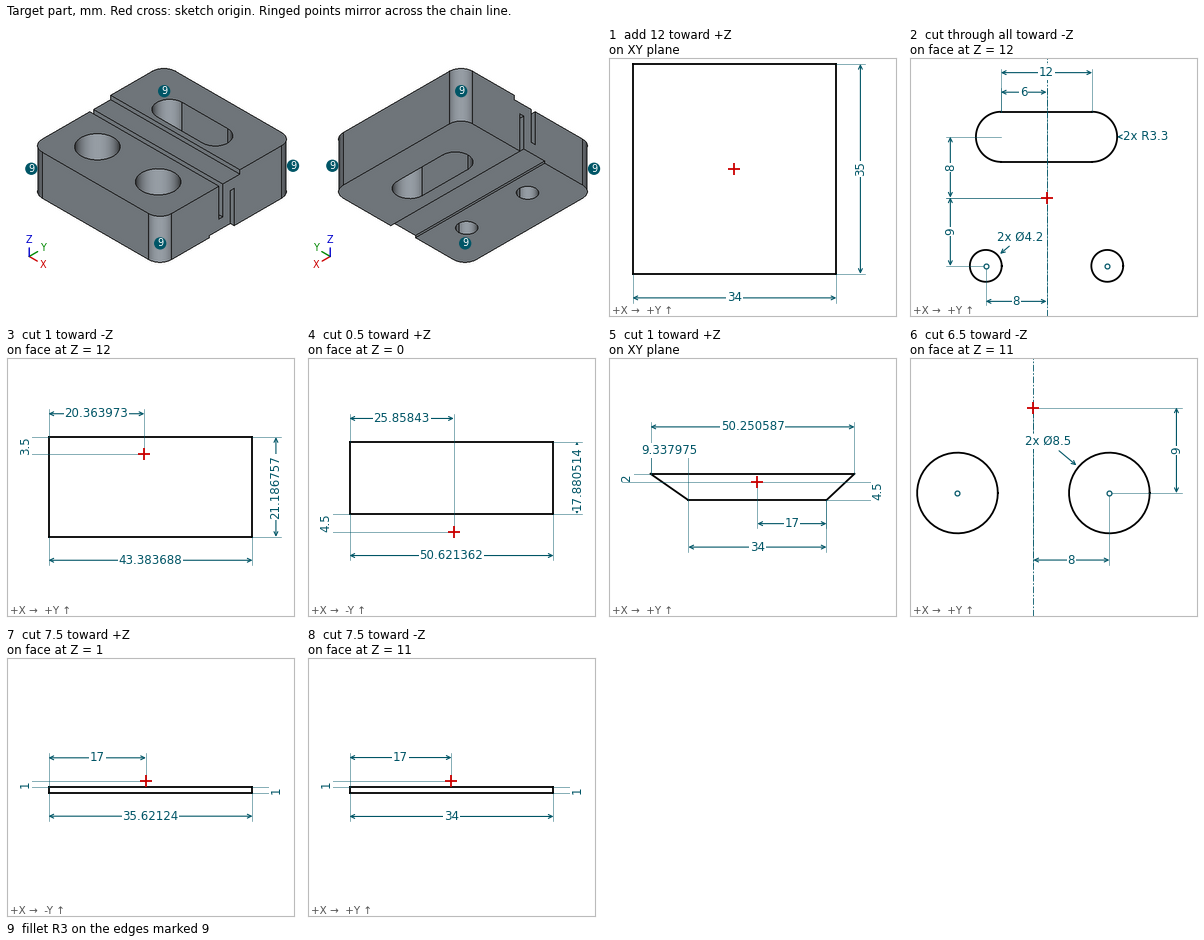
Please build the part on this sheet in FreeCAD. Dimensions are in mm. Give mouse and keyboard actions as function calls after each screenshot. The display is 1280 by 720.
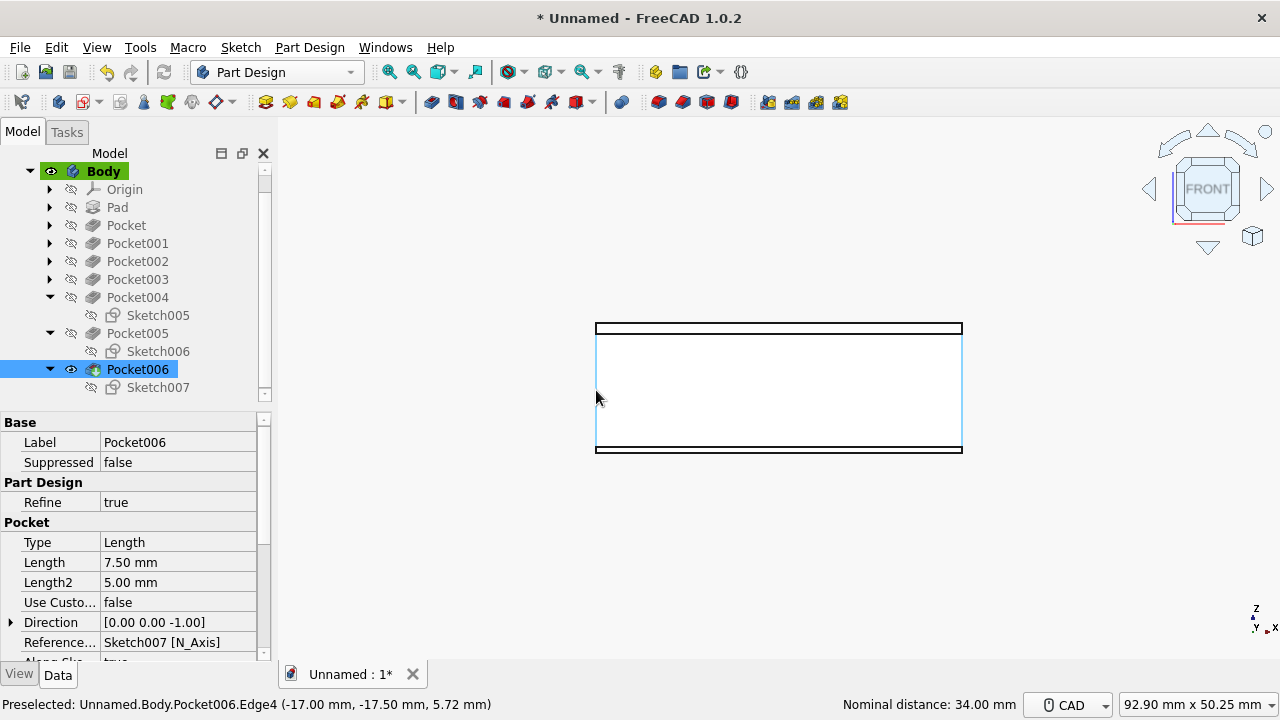
key(3)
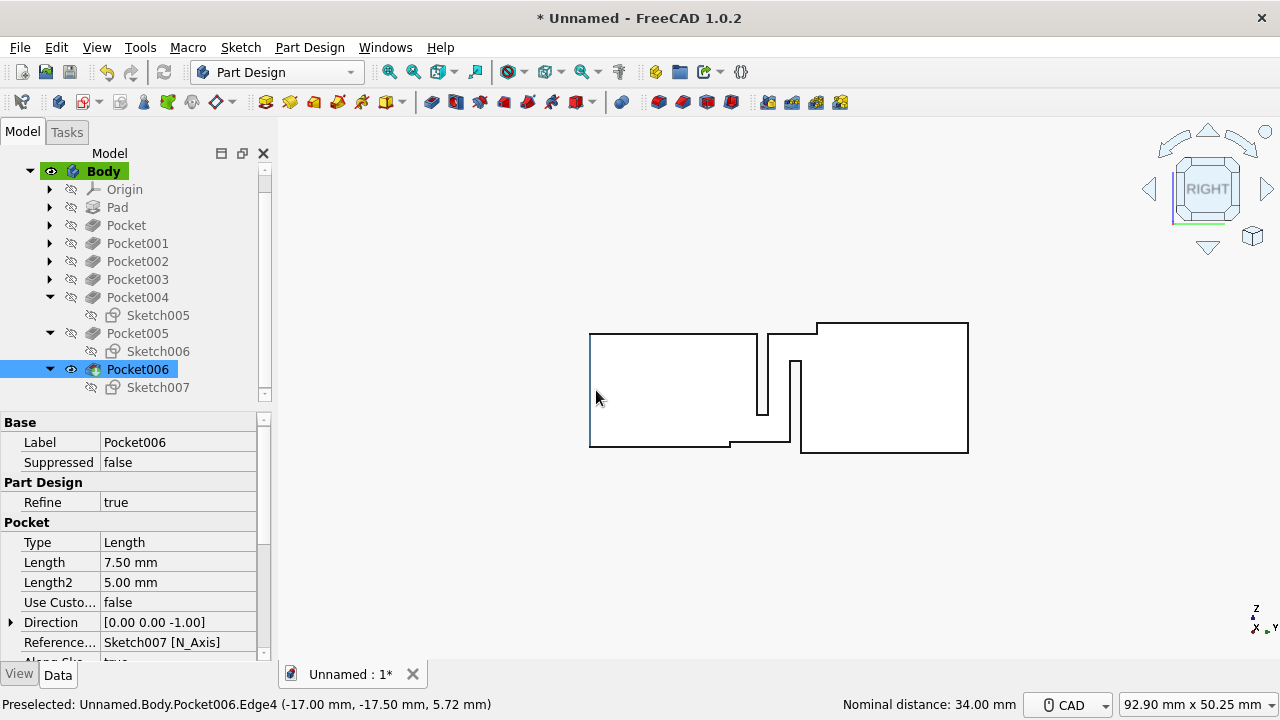
key(v)
key(f)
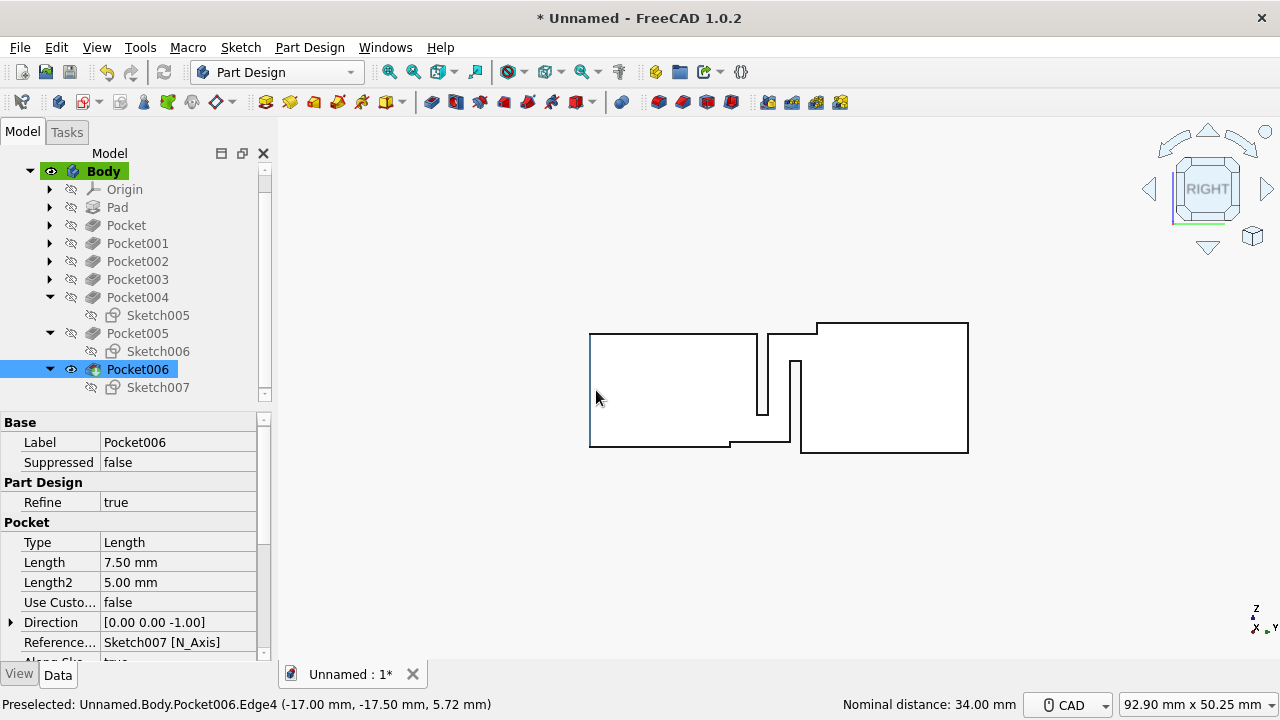
click(968, 387, ctrl)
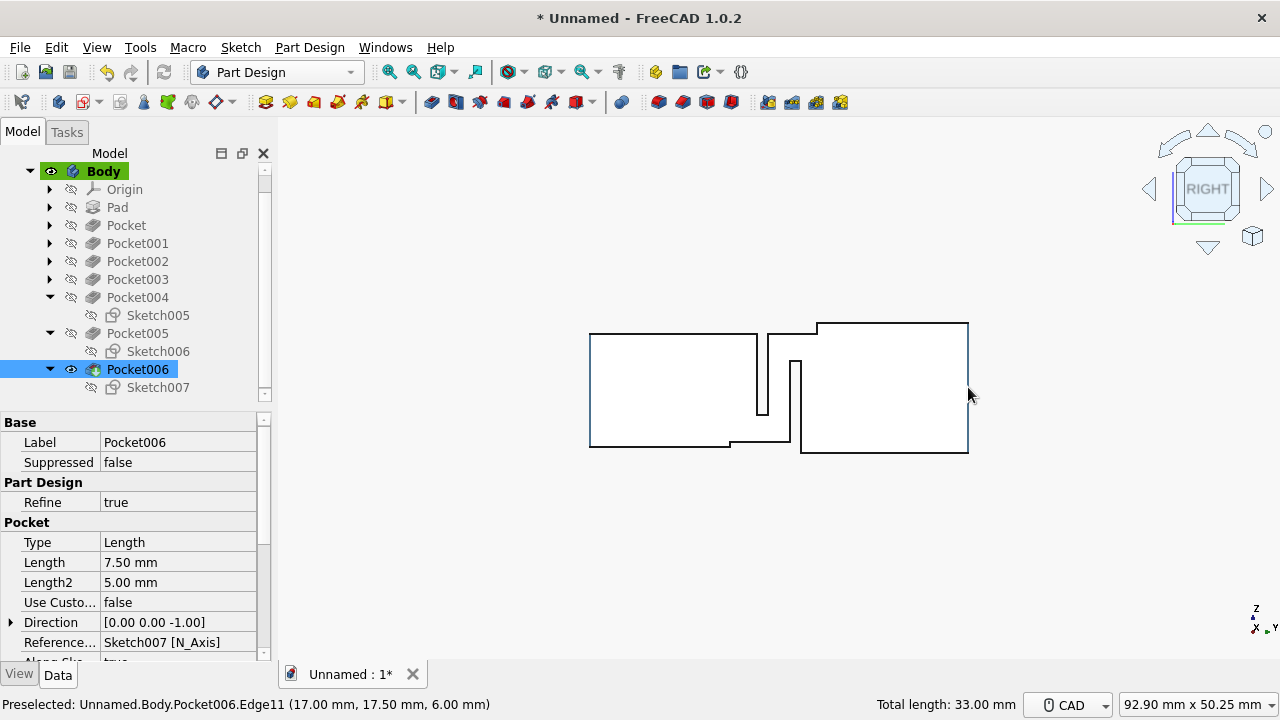
key(5)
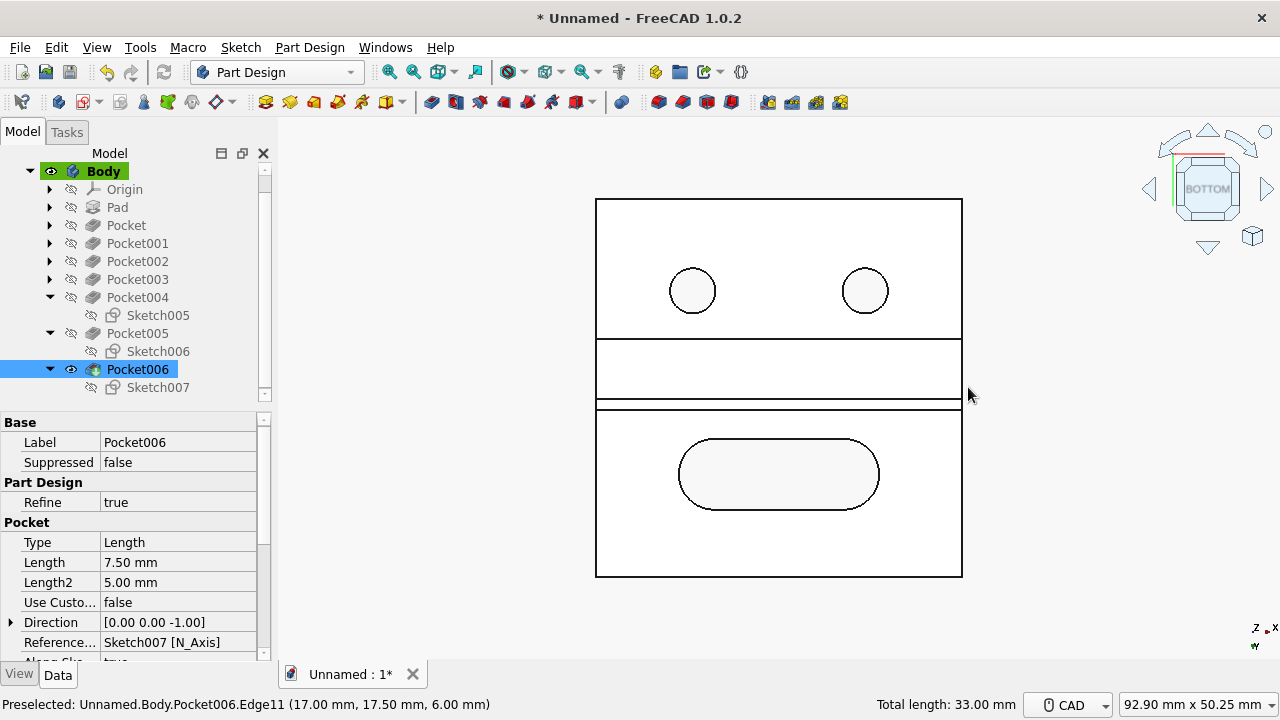
key(4)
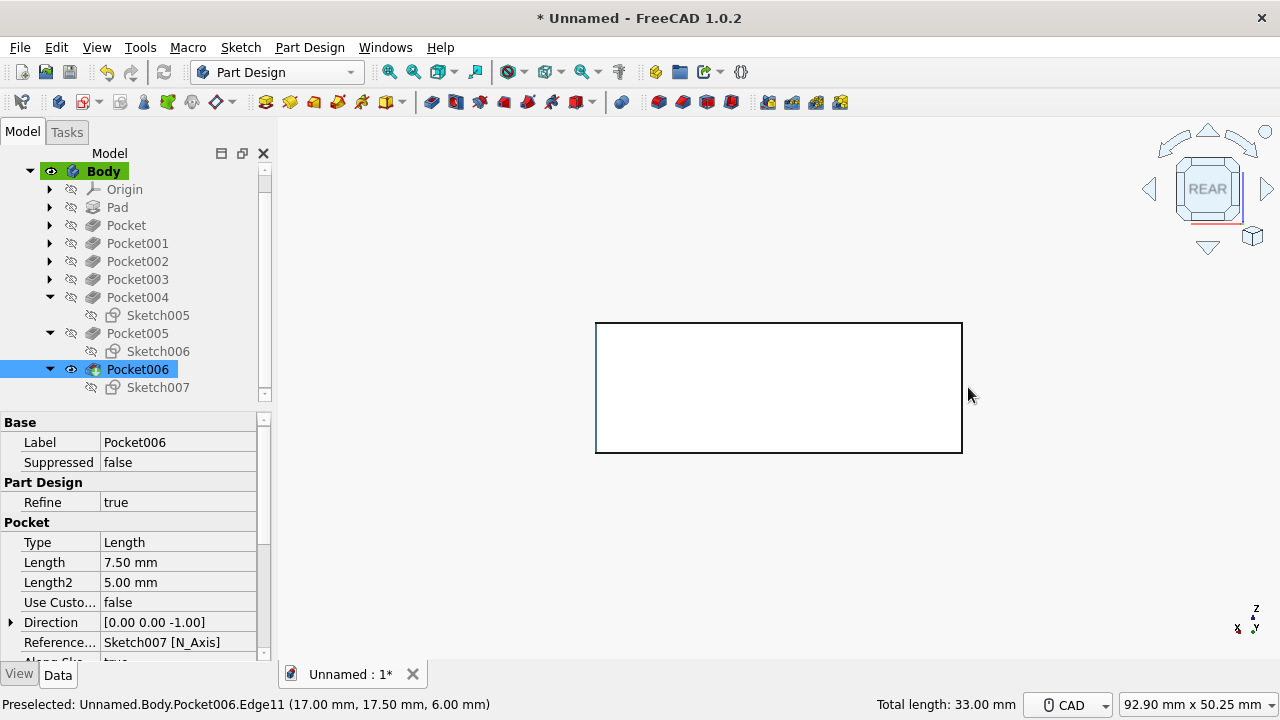
key(v)
key(f)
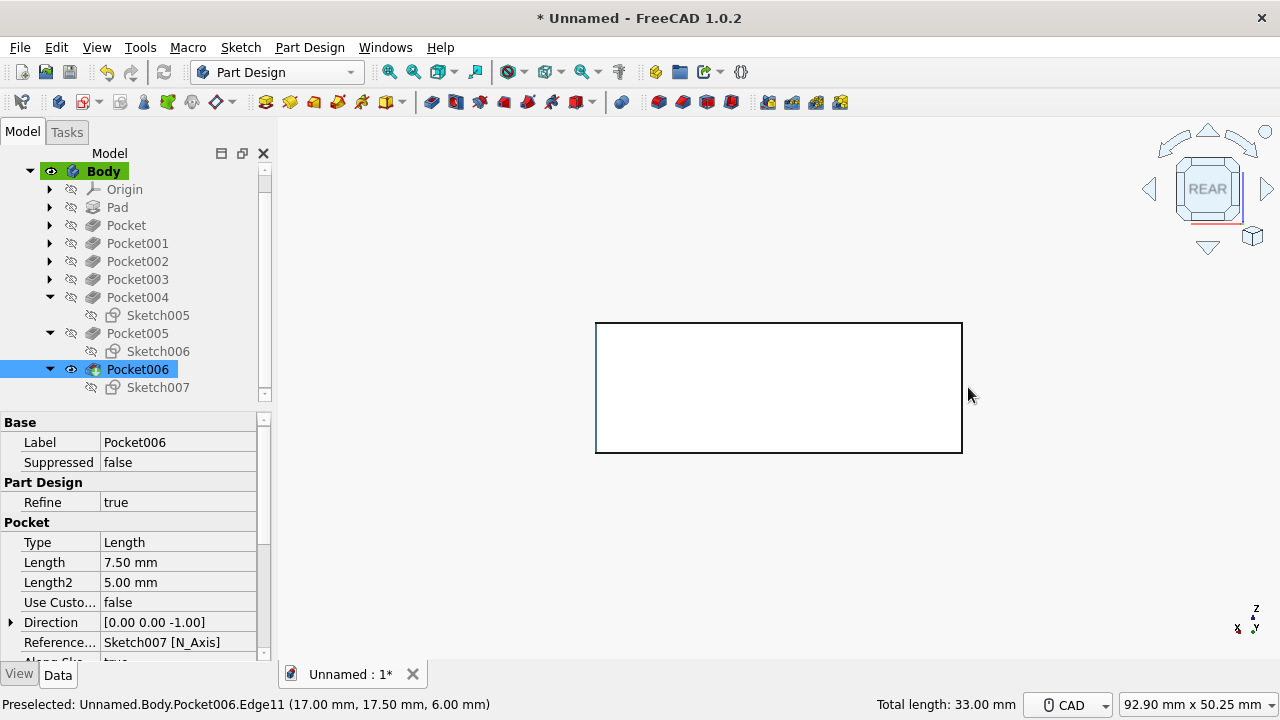
click(962, 387, ctrl)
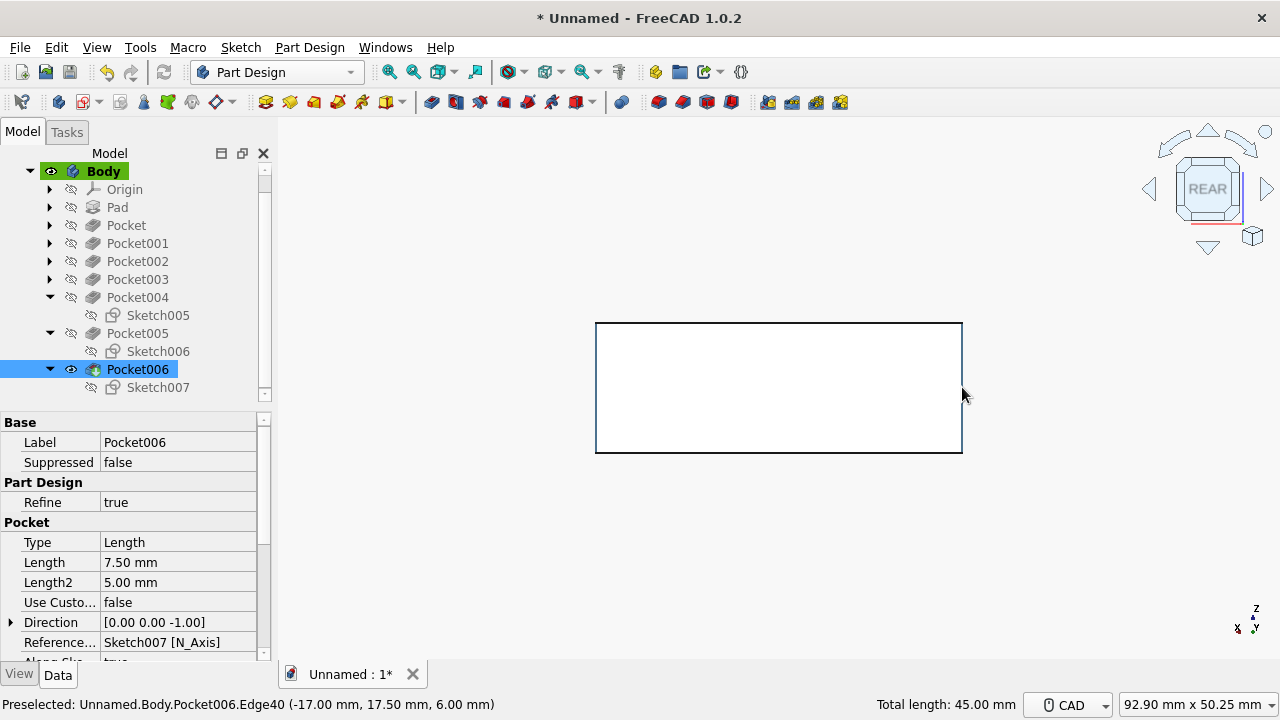
click(660, 102)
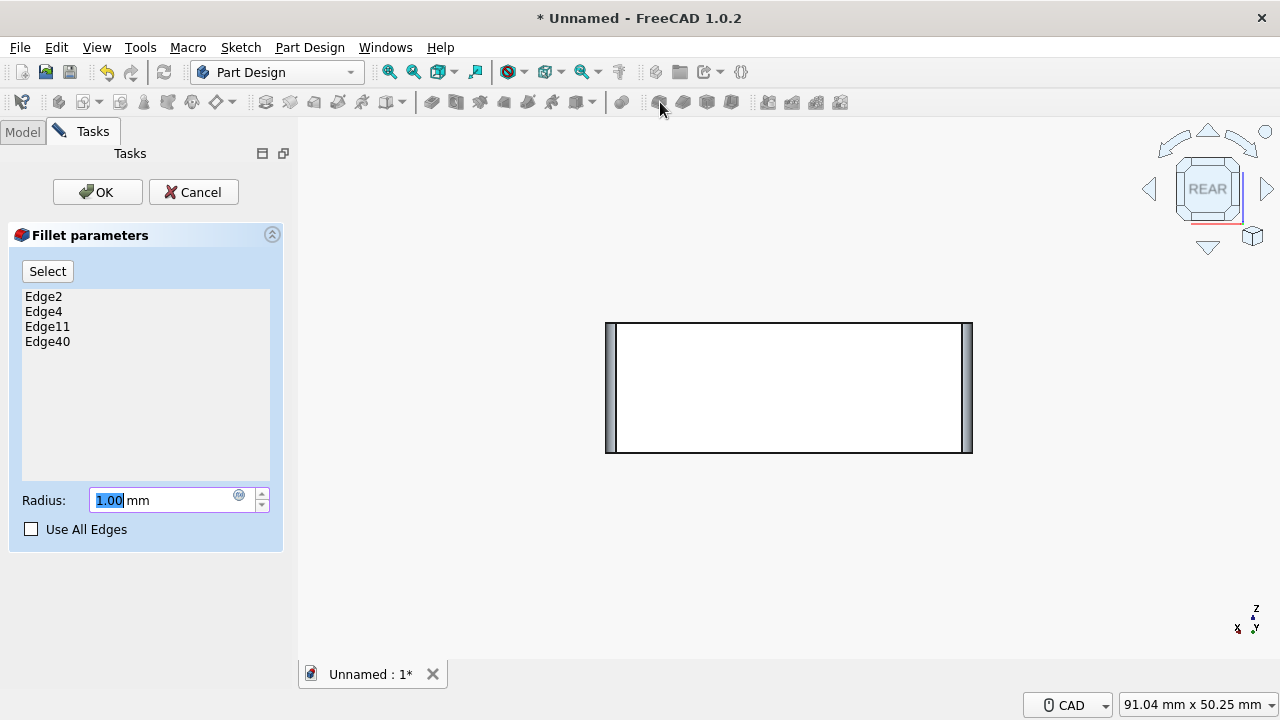
text(3)
key(Tab)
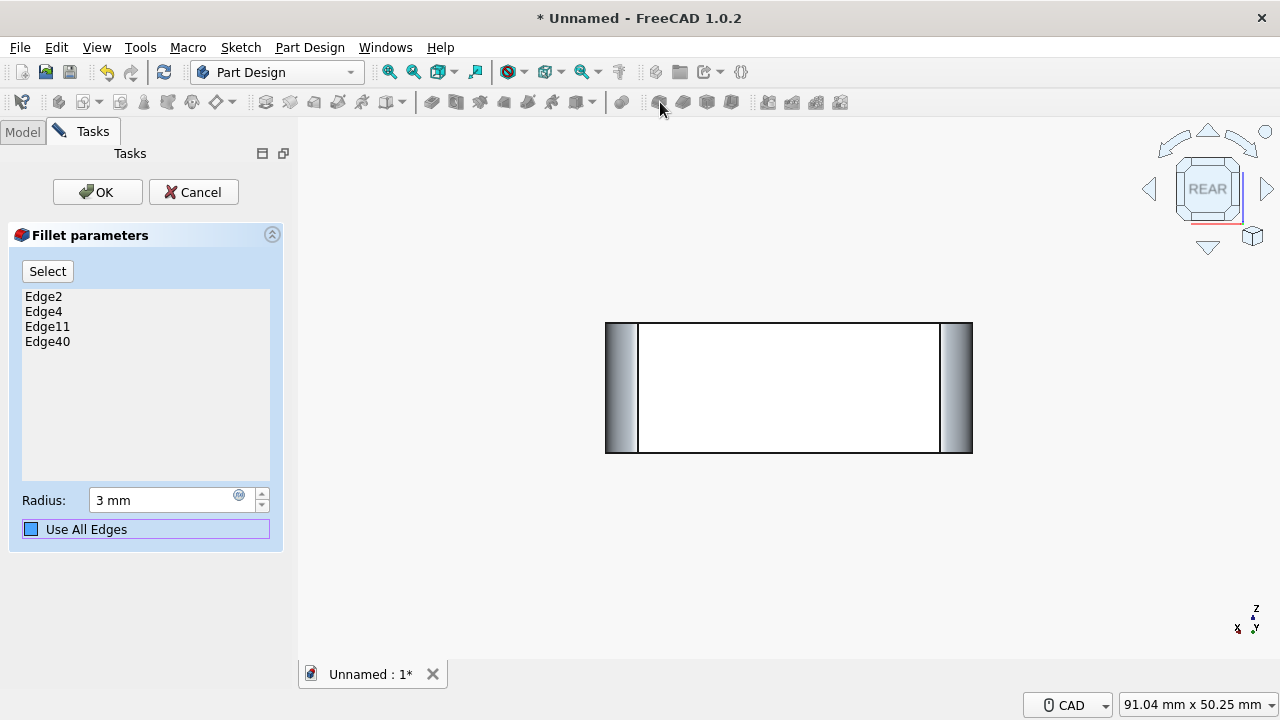
click(98, 192)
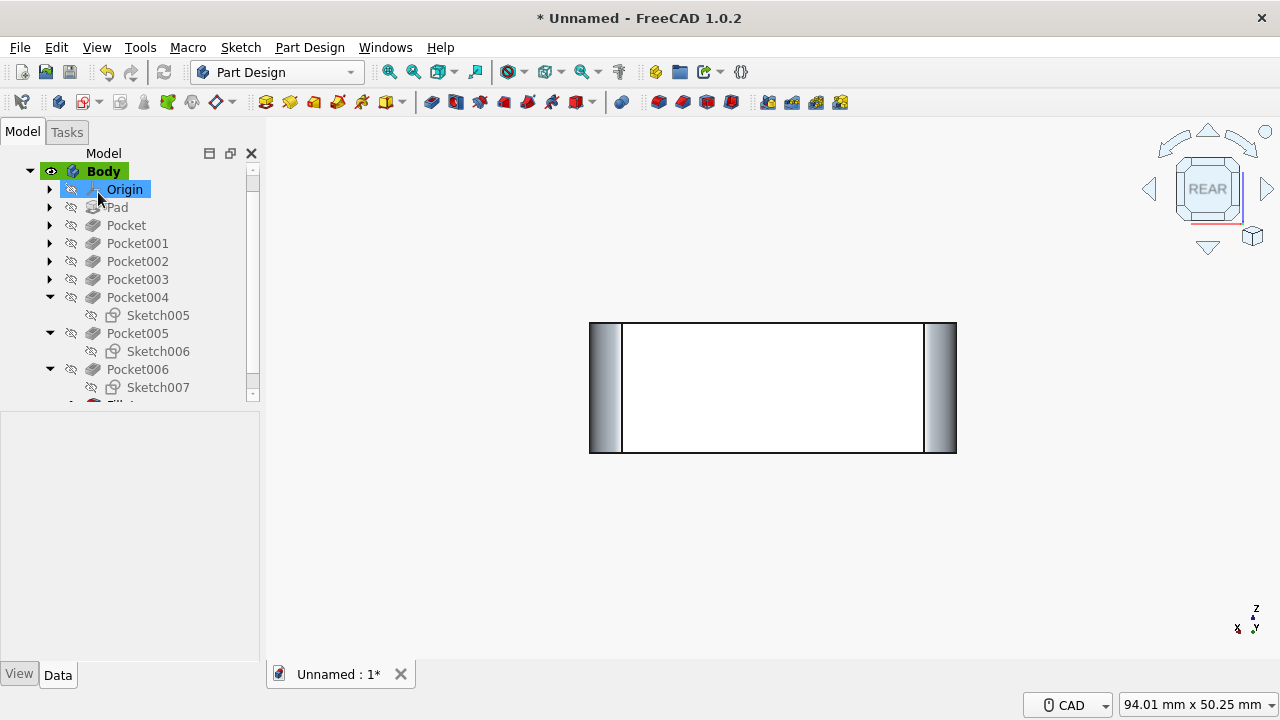
key(0)